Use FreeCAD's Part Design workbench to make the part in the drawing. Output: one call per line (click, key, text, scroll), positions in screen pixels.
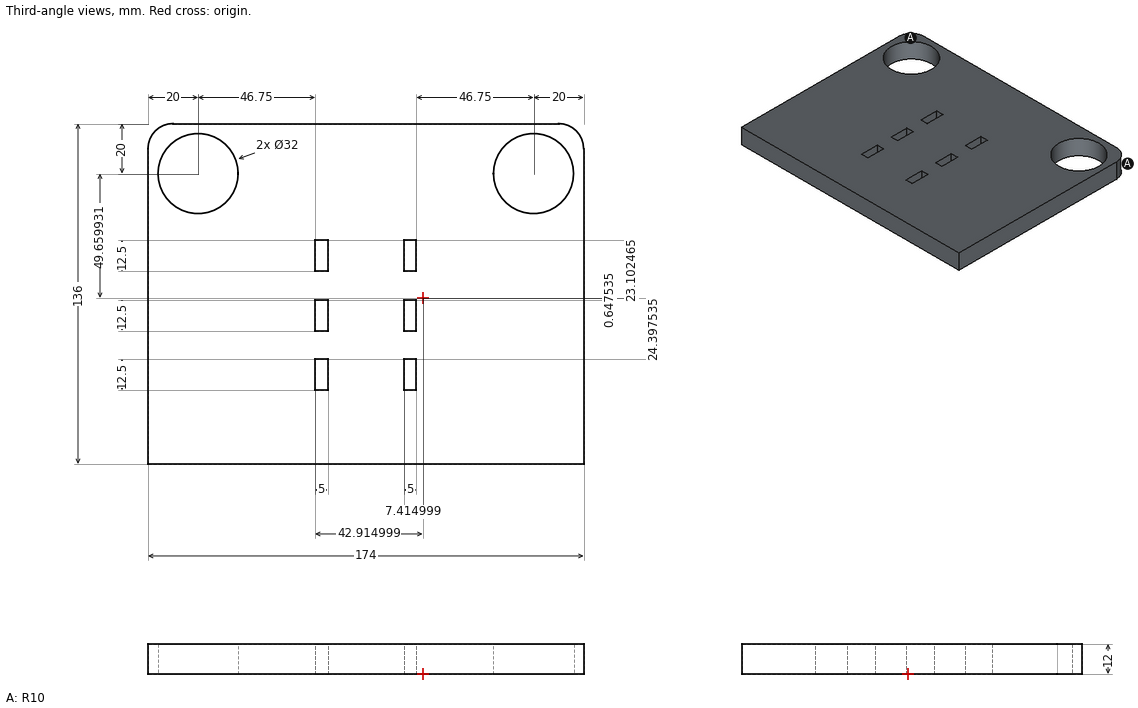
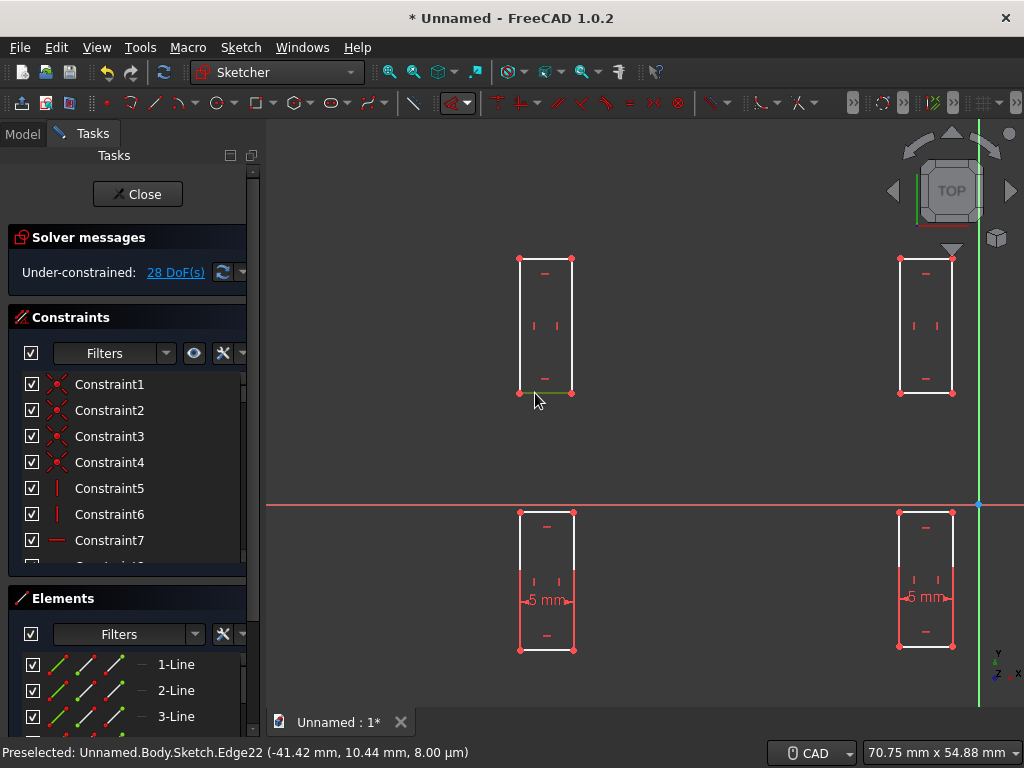
click(470, 104)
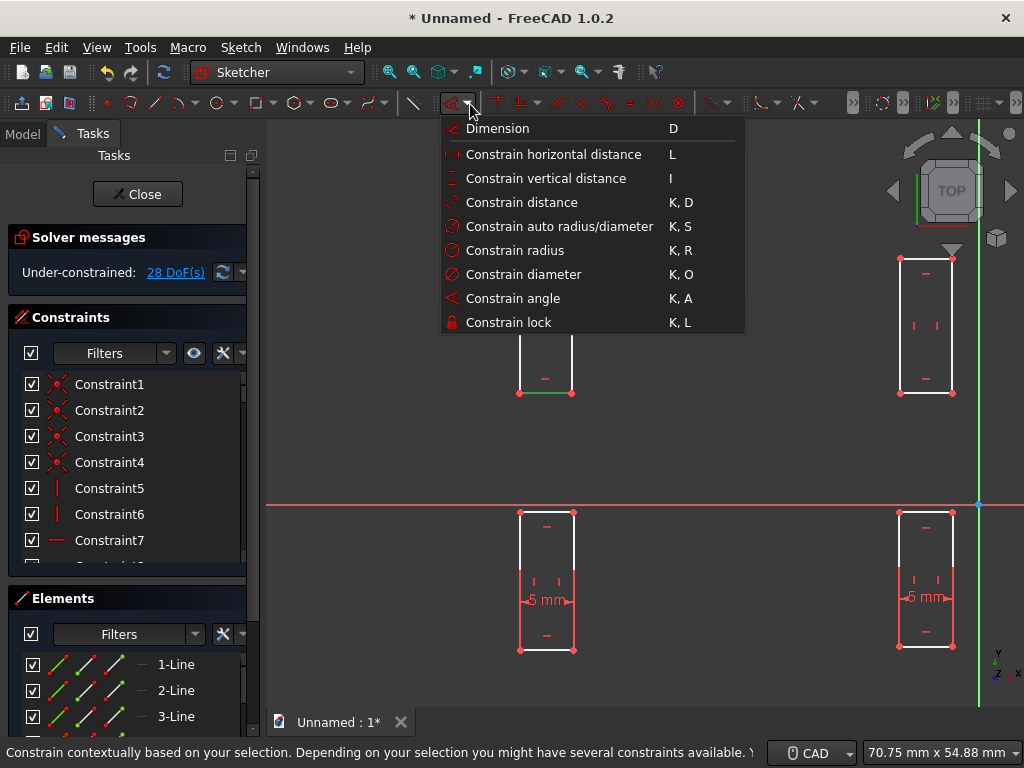
click(593, 154)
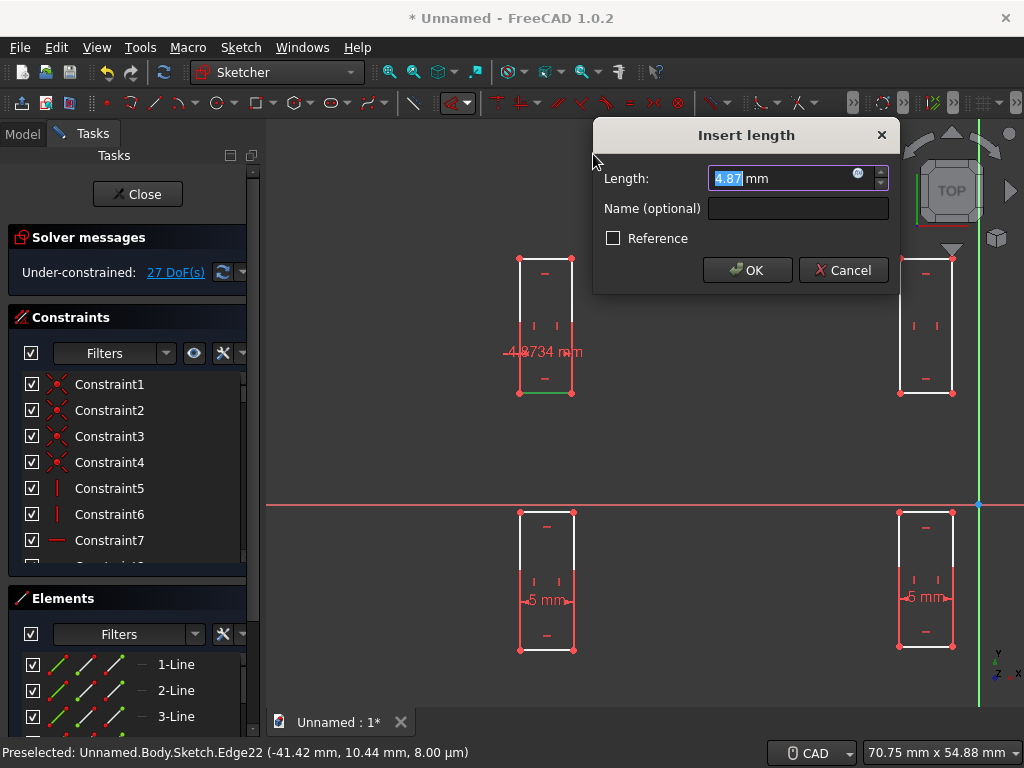
text(5)
key(Return)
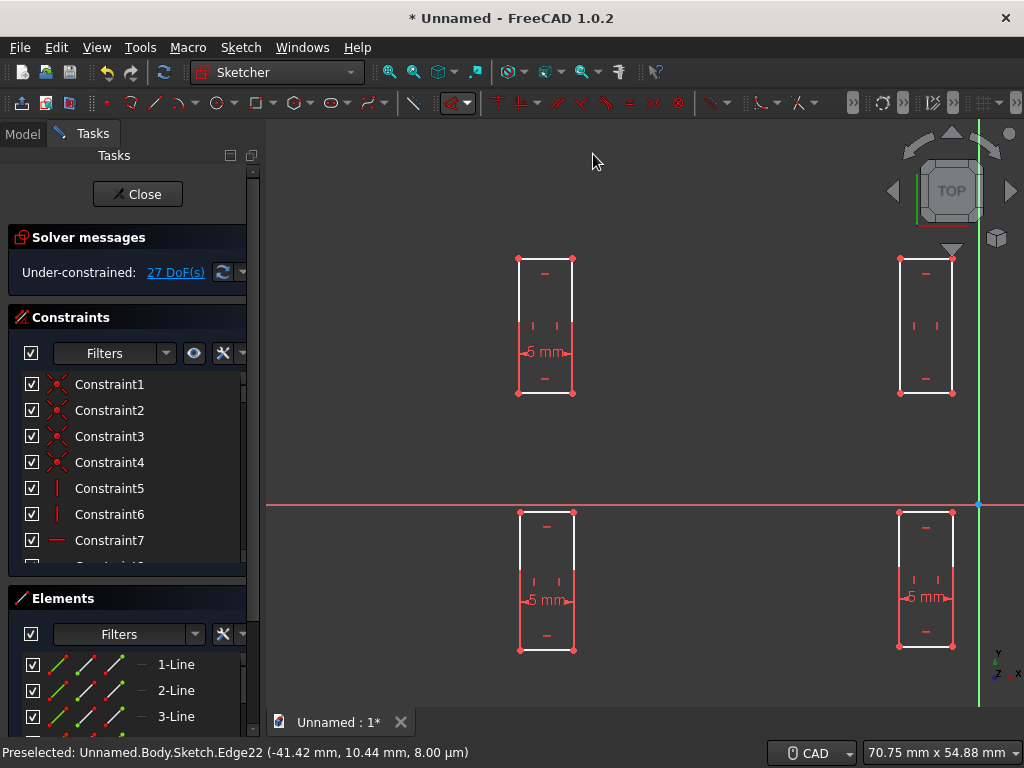
scroll(536, 394, down, 8)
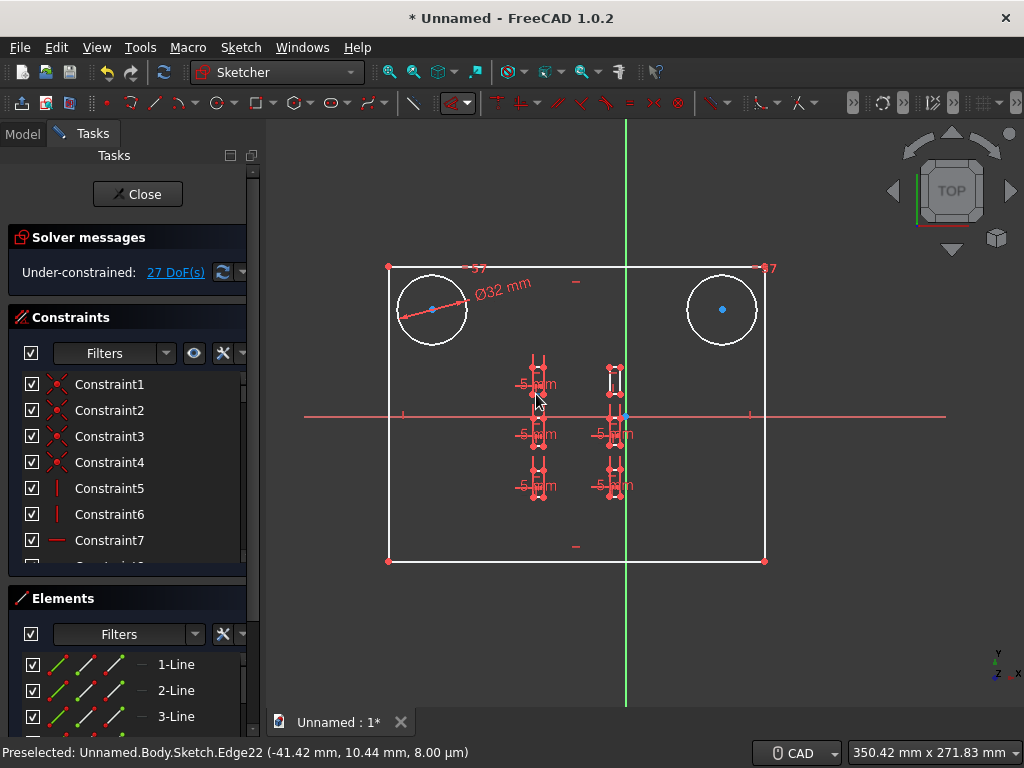
scroll(613, 394, up, 8)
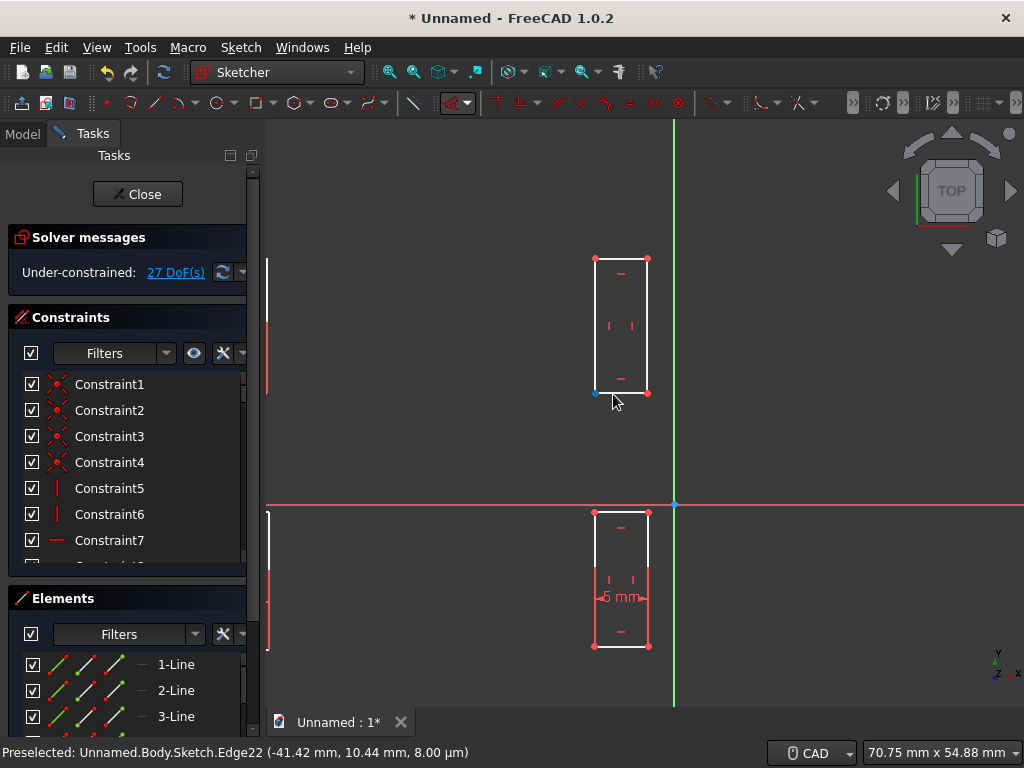
click(611, 393)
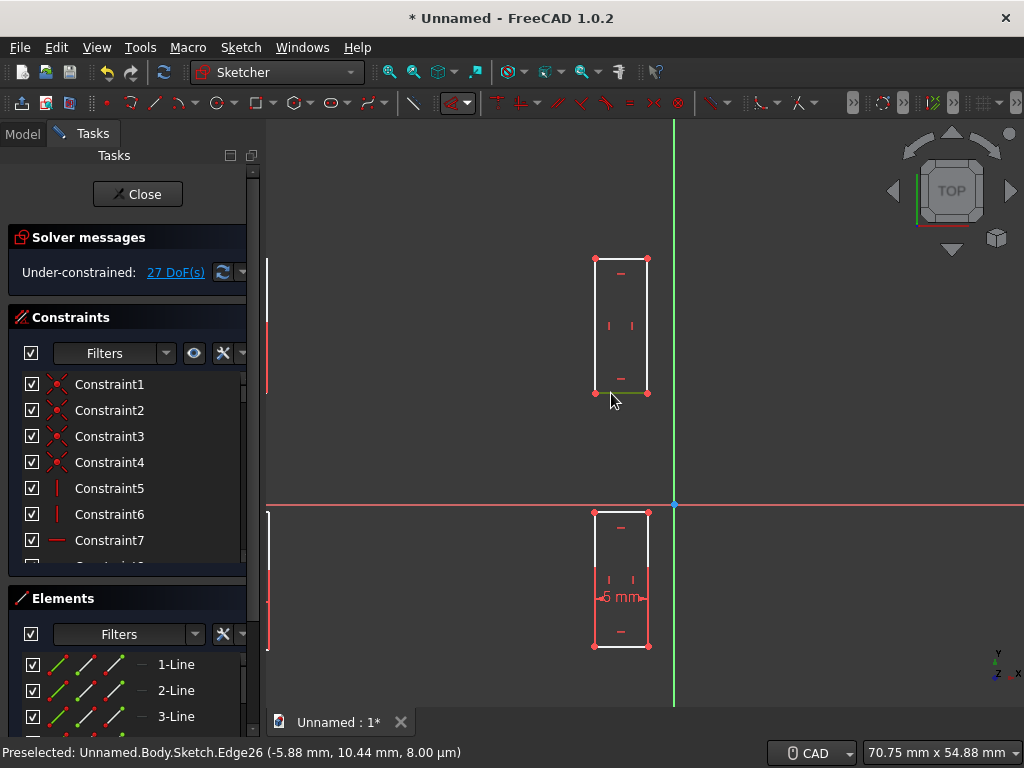
click(470, 104)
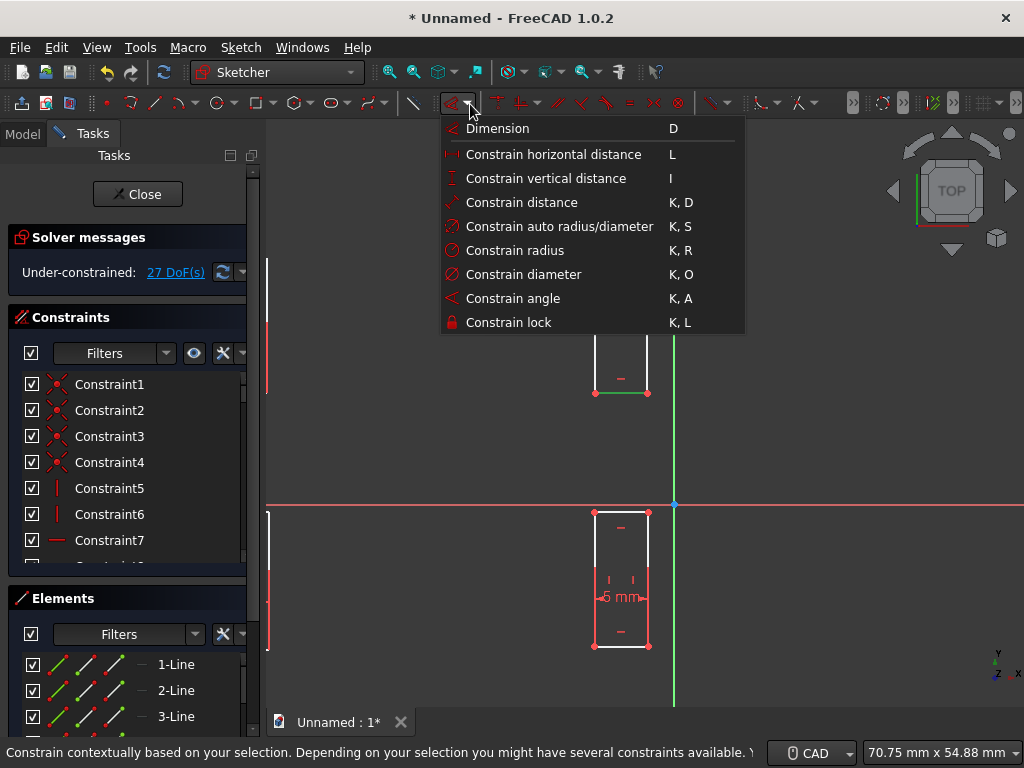
click(593, 154)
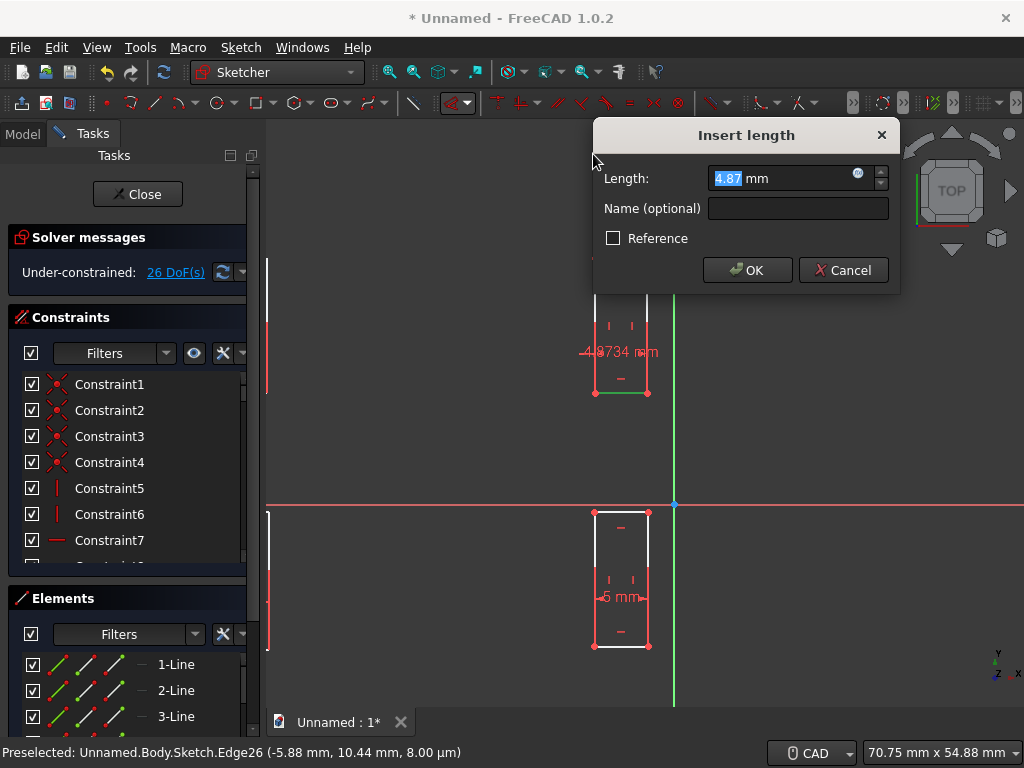
text(5)
key(Return)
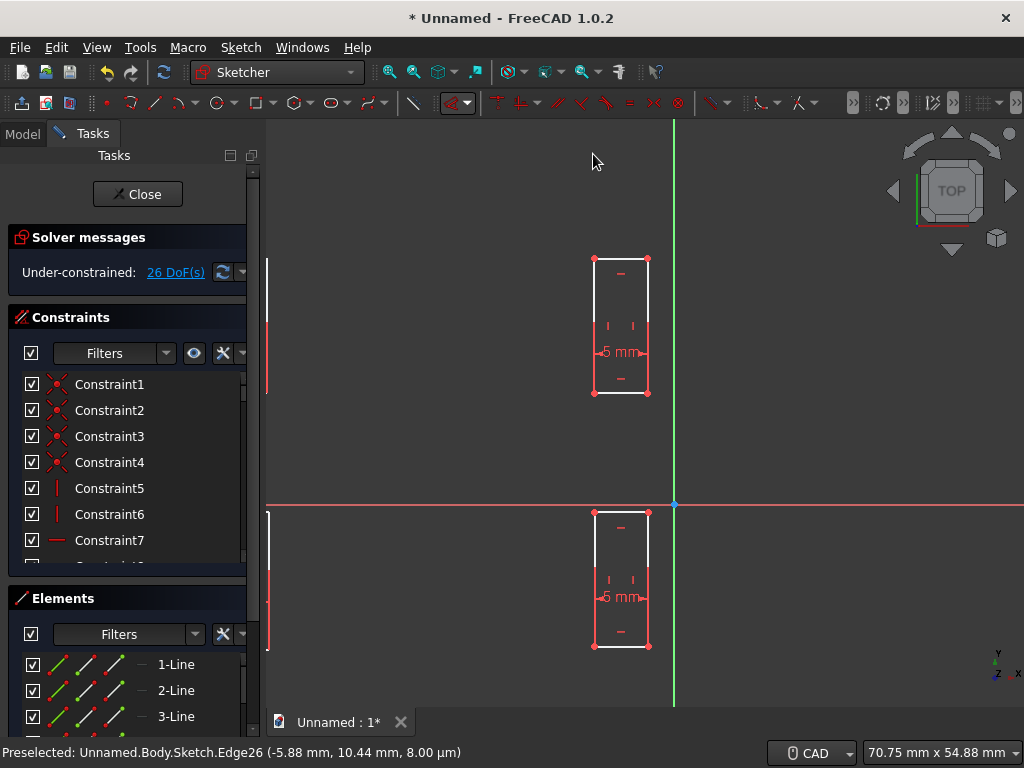
scroll(613, 394, down, 8)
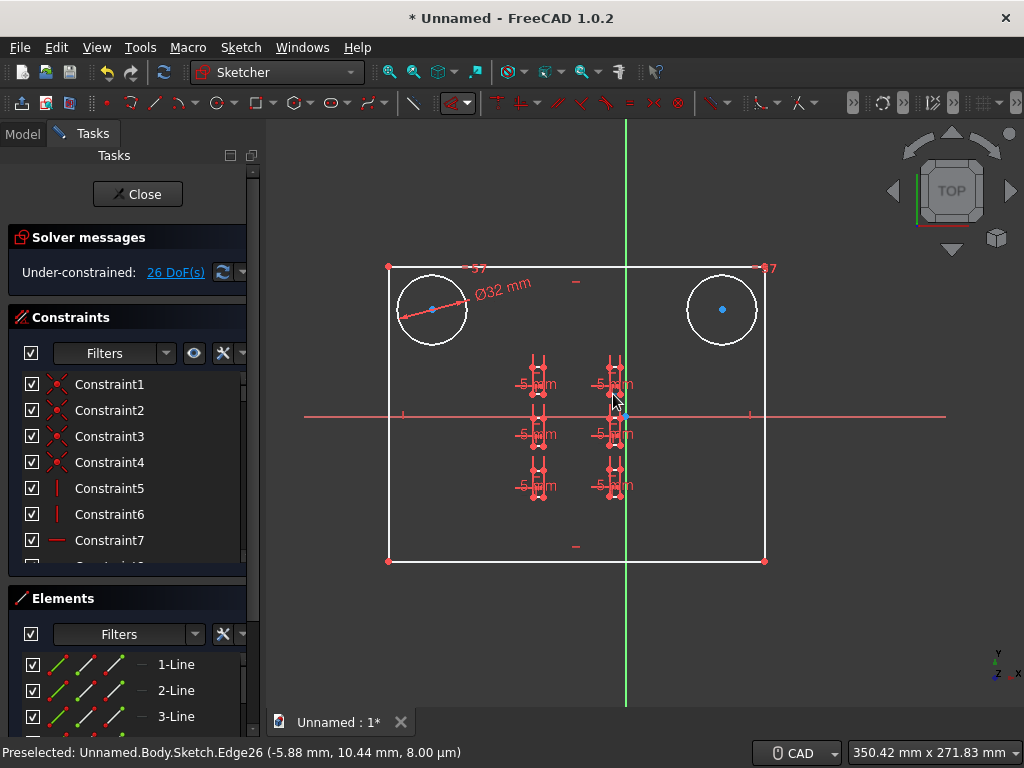
click(389, 355)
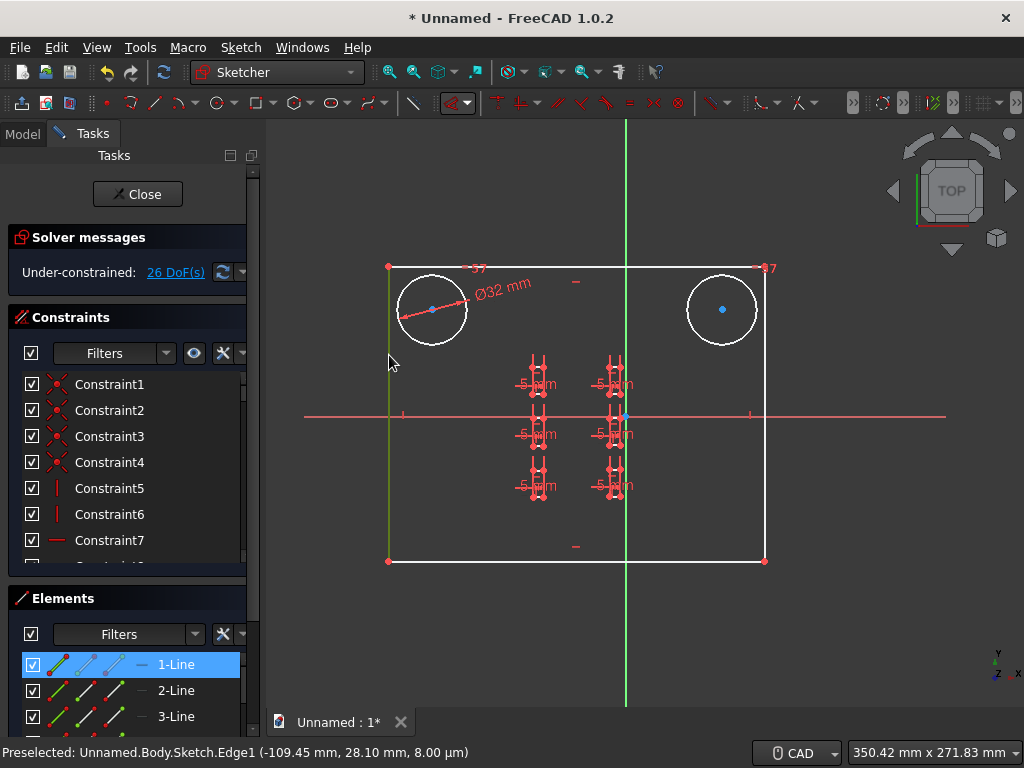
click(470, 104)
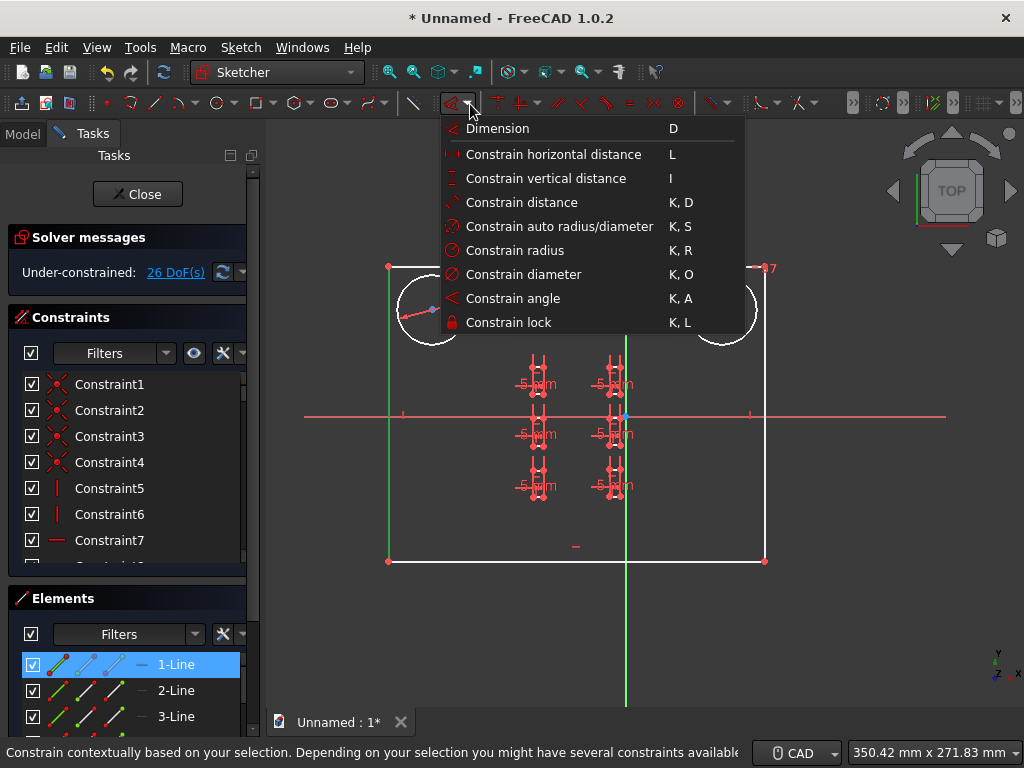
click(593, 178)